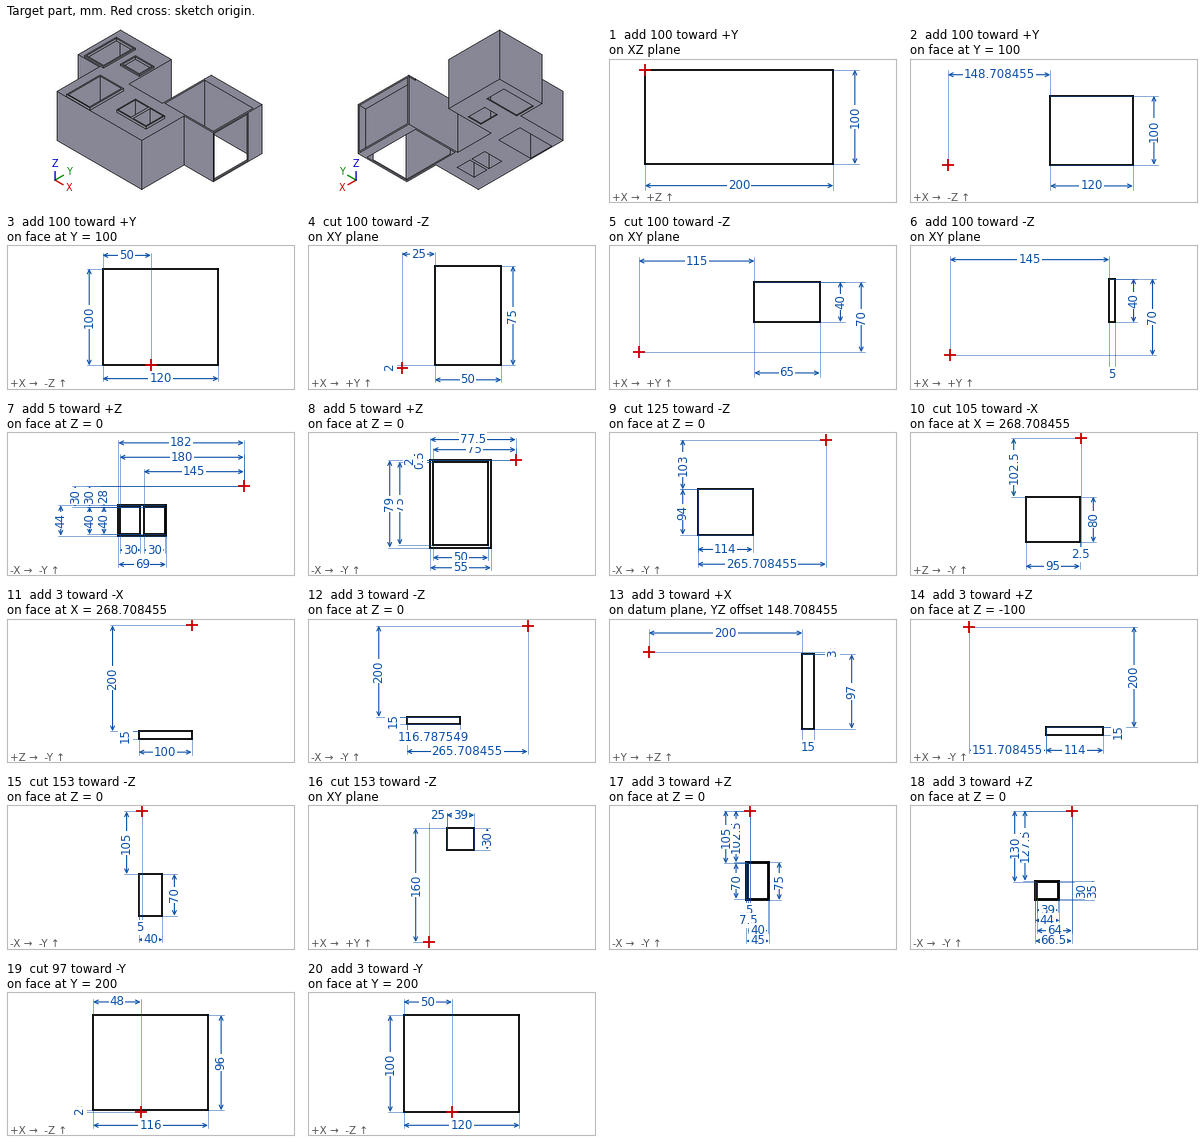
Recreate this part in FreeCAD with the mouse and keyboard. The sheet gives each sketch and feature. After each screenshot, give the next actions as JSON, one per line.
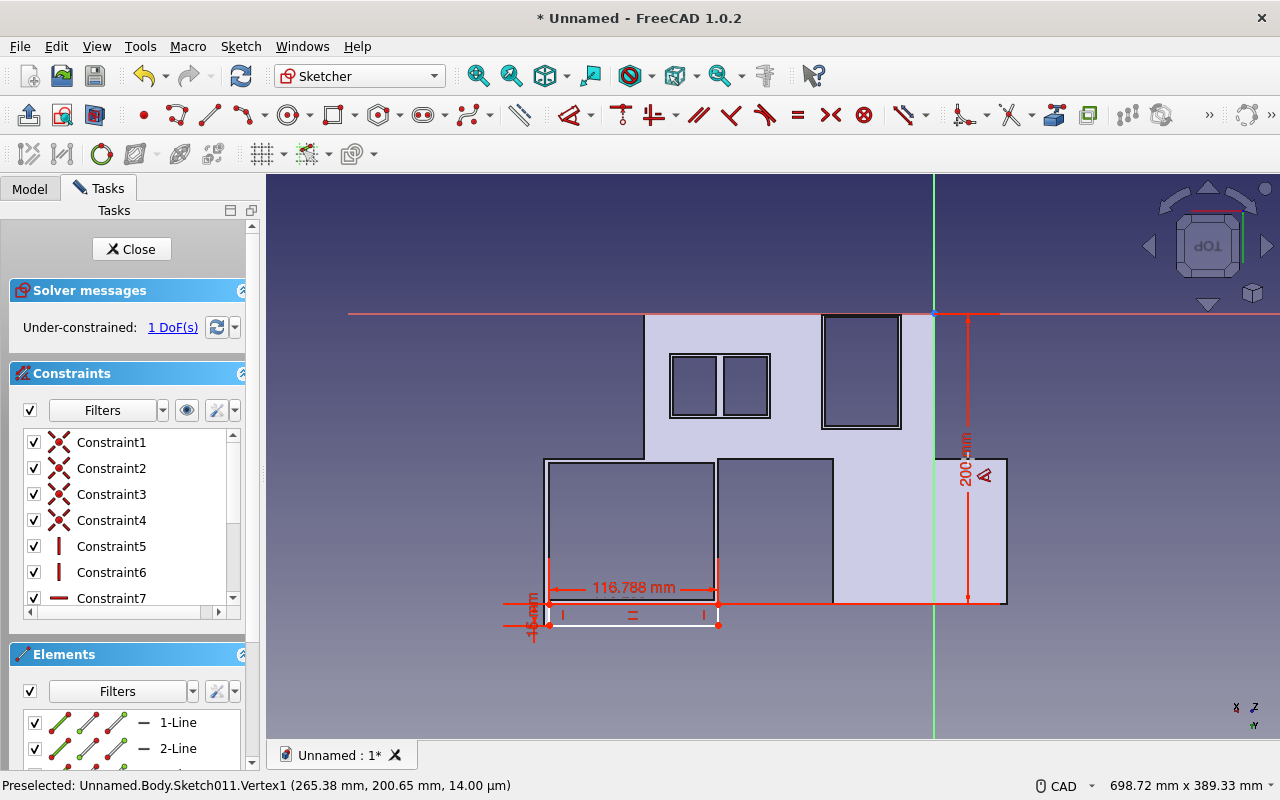
{"action": "left_click", "coordinate": [549, 604]}
{"action": "left_click", "coordinate": [742, 280]}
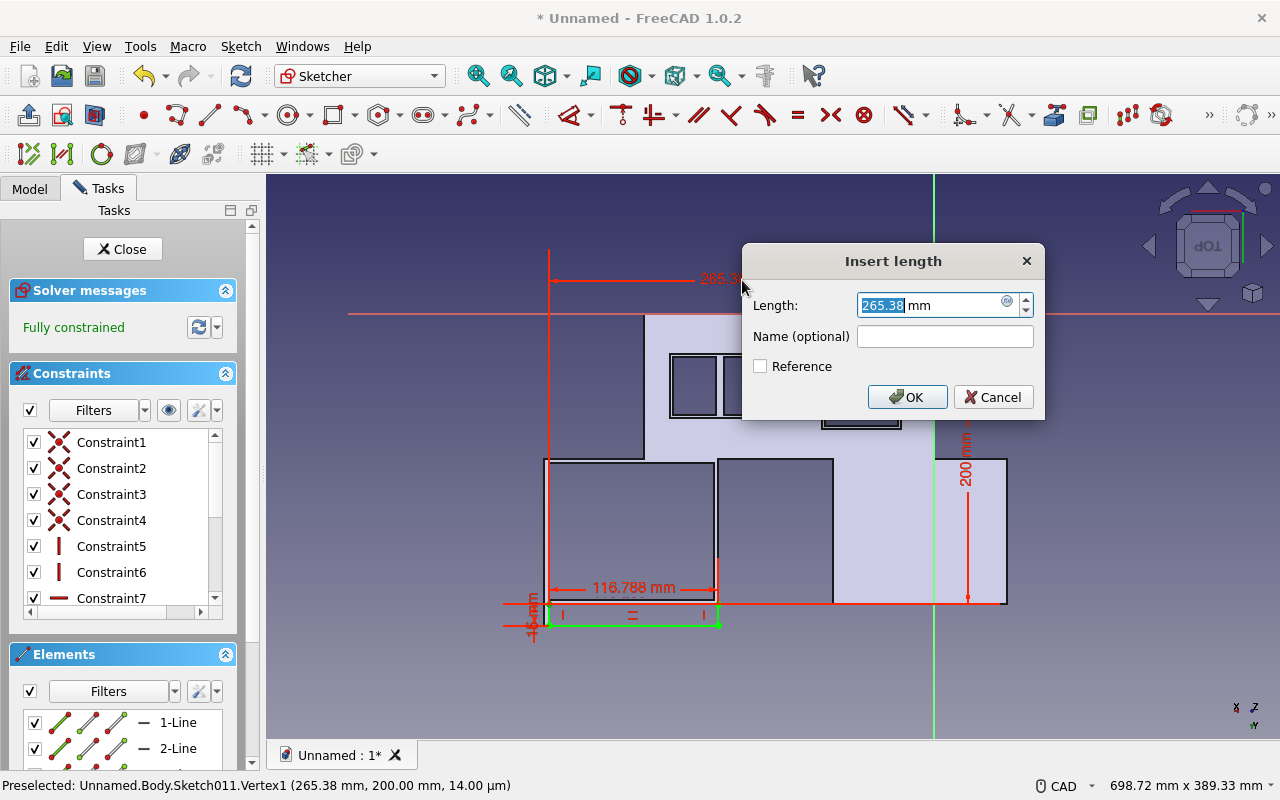
{"action": "type", "text": "265.708455"}
{"action": "key", "text": "Return"}
{"action": "key", "text": "Escape"}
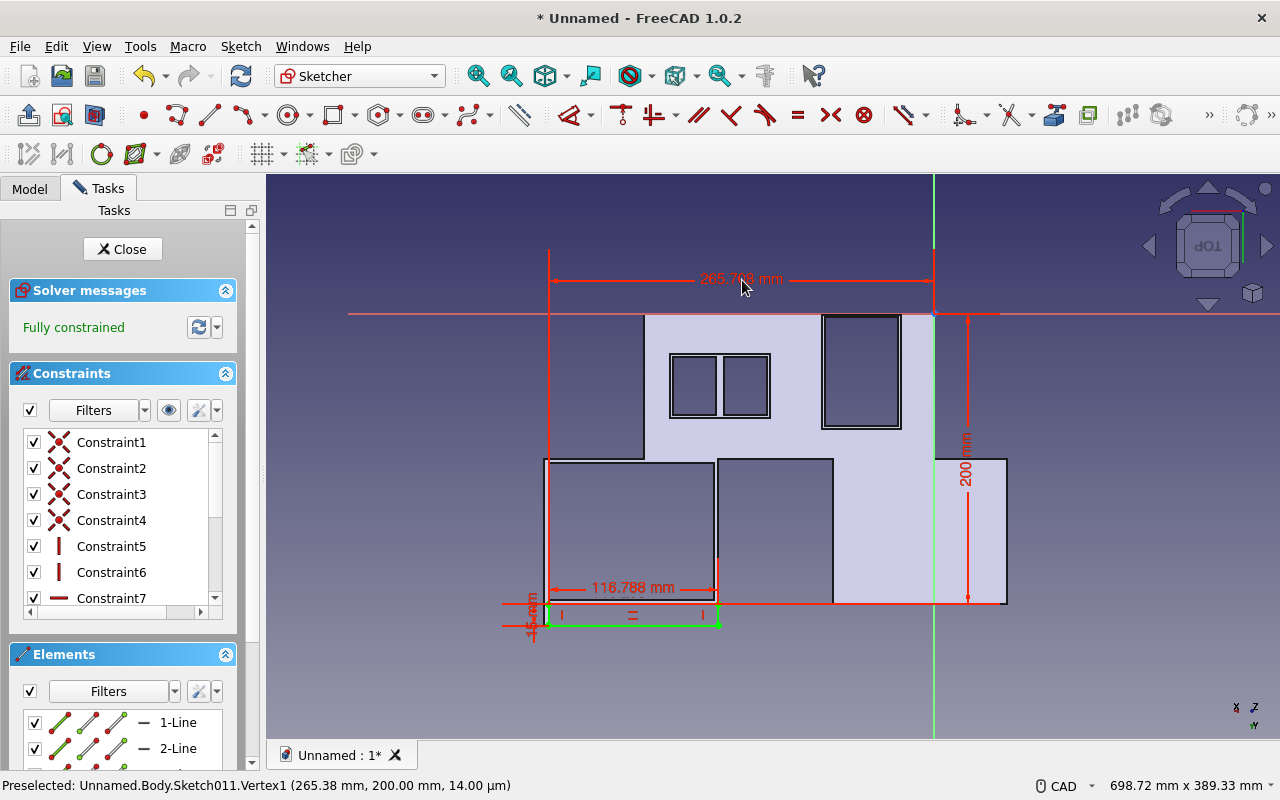
{"action": "left_click", "coordinate": [123, 249]}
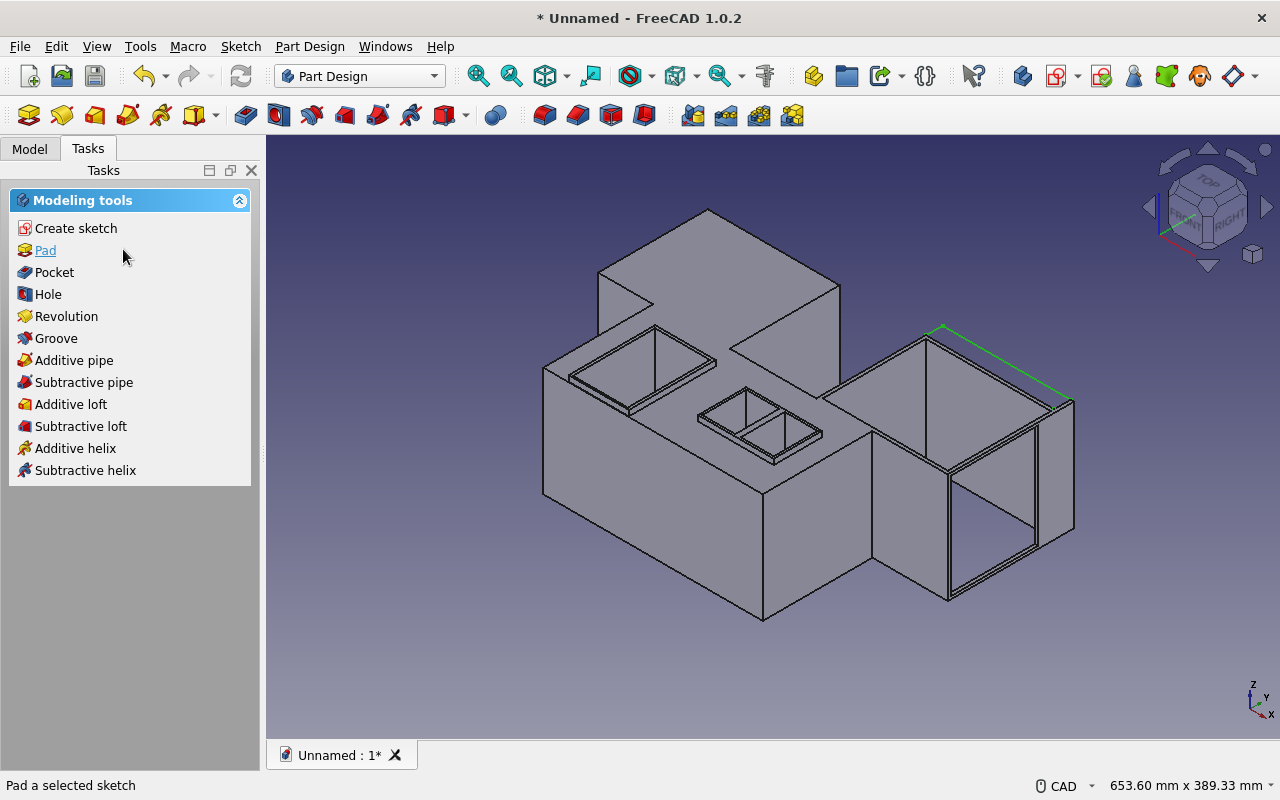
{"action": "left_click", "coordinate": [29, 116]}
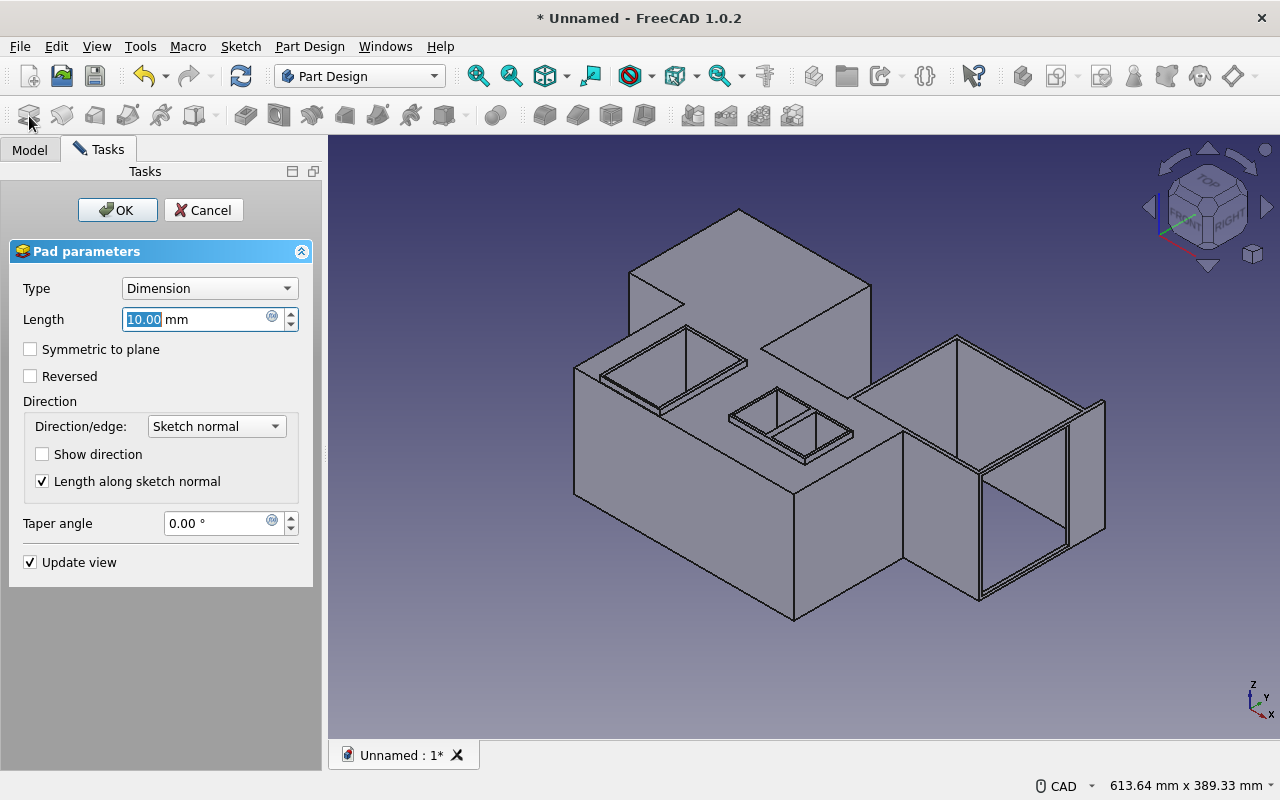
{"action": "type", "text": "3"}
{"action": "key", "text": "Tab"}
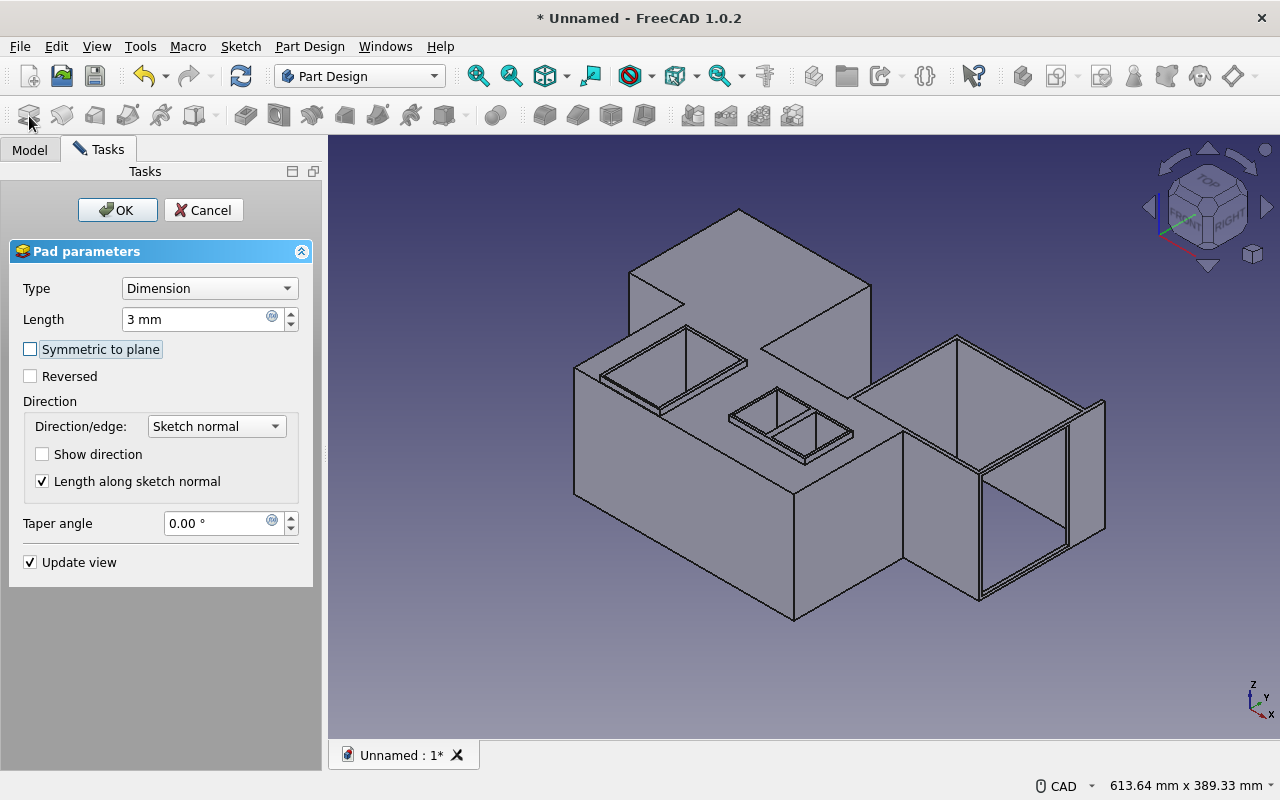
{"action": "left_click", "coordinate": [31, 376]}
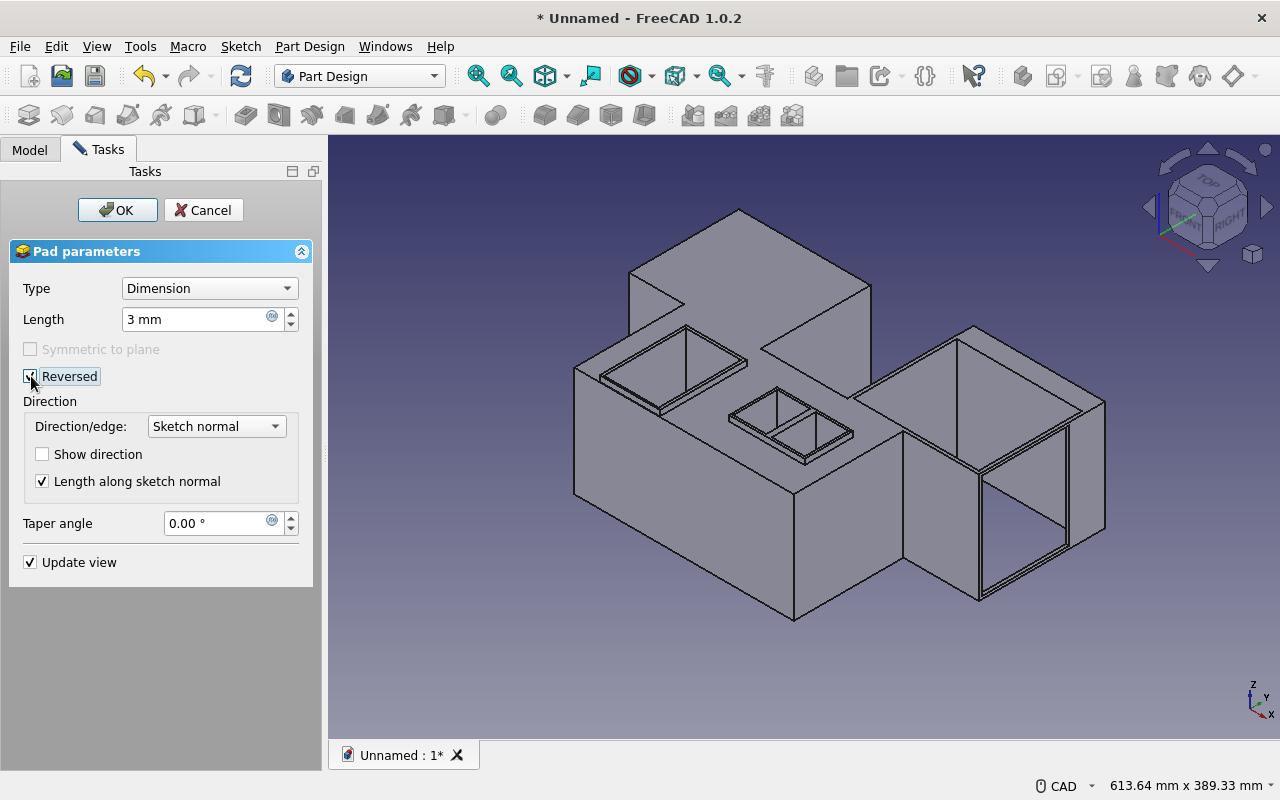
{"action": "left_click", "coordinate": [118, 210]}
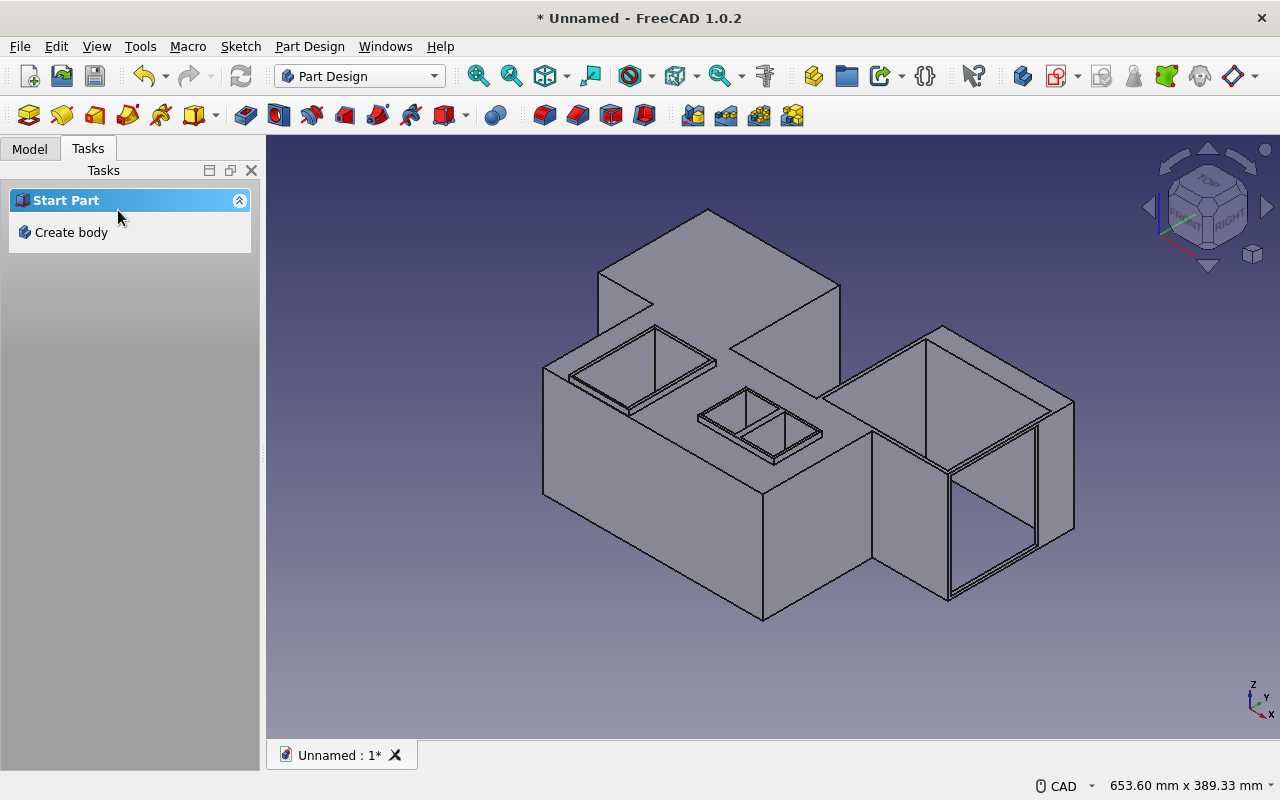
{"action": "left_click", "coordinate": [30, 148]}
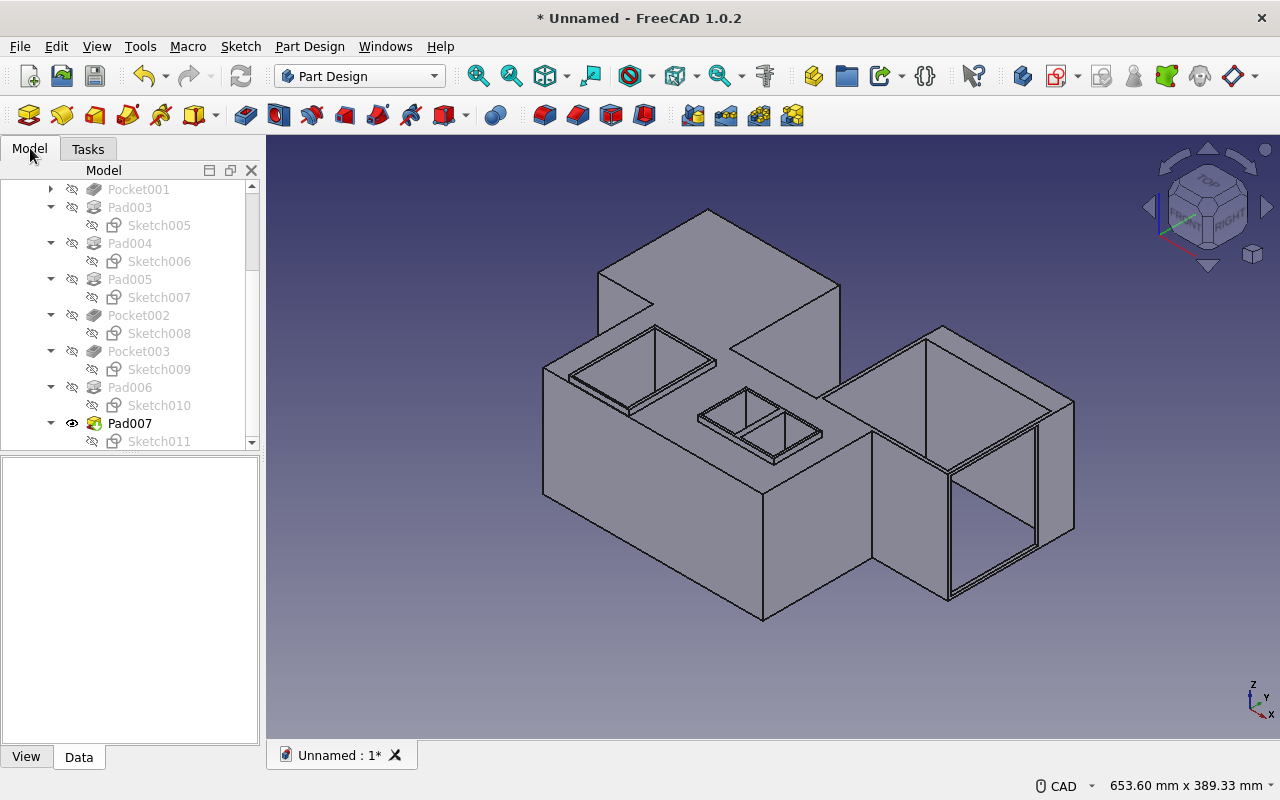
{"action": "scroll", "coordinate": [141, 311], "scroll_direction": "down", "scroll_amount": 3}